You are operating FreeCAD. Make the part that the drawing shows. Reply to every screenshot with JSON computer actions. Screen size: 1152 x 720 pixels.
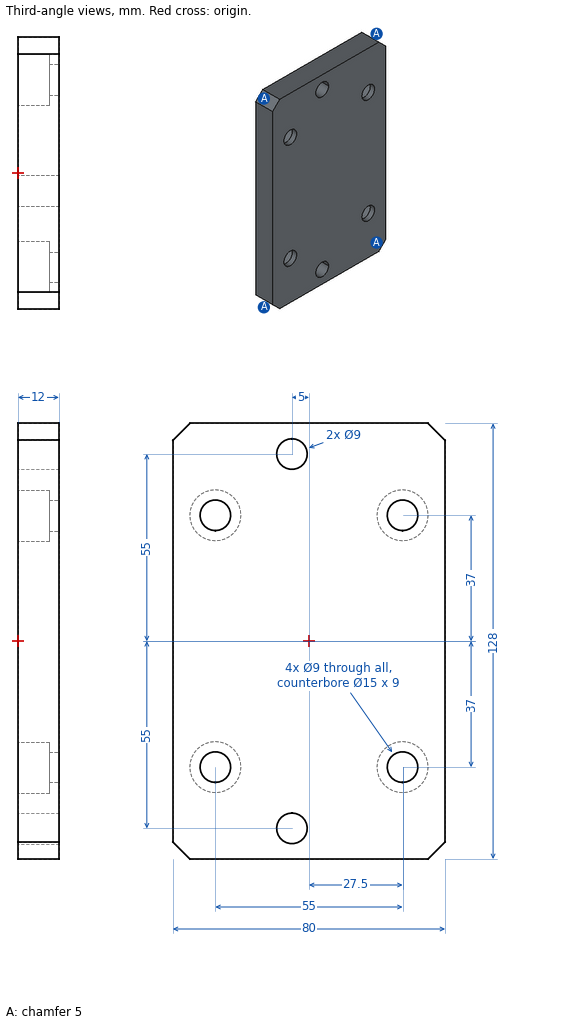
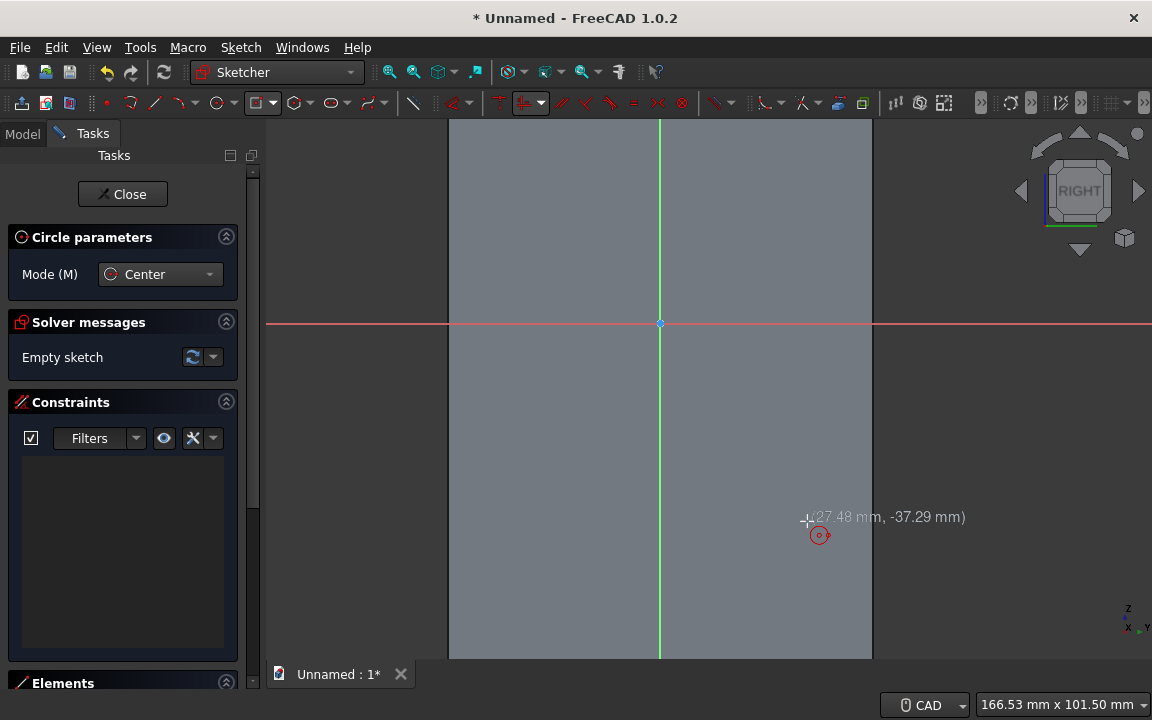
{"action": "left_click", "coordinate": [807, 521]}
{"action": "left_click", "coordinate": [824, 504]}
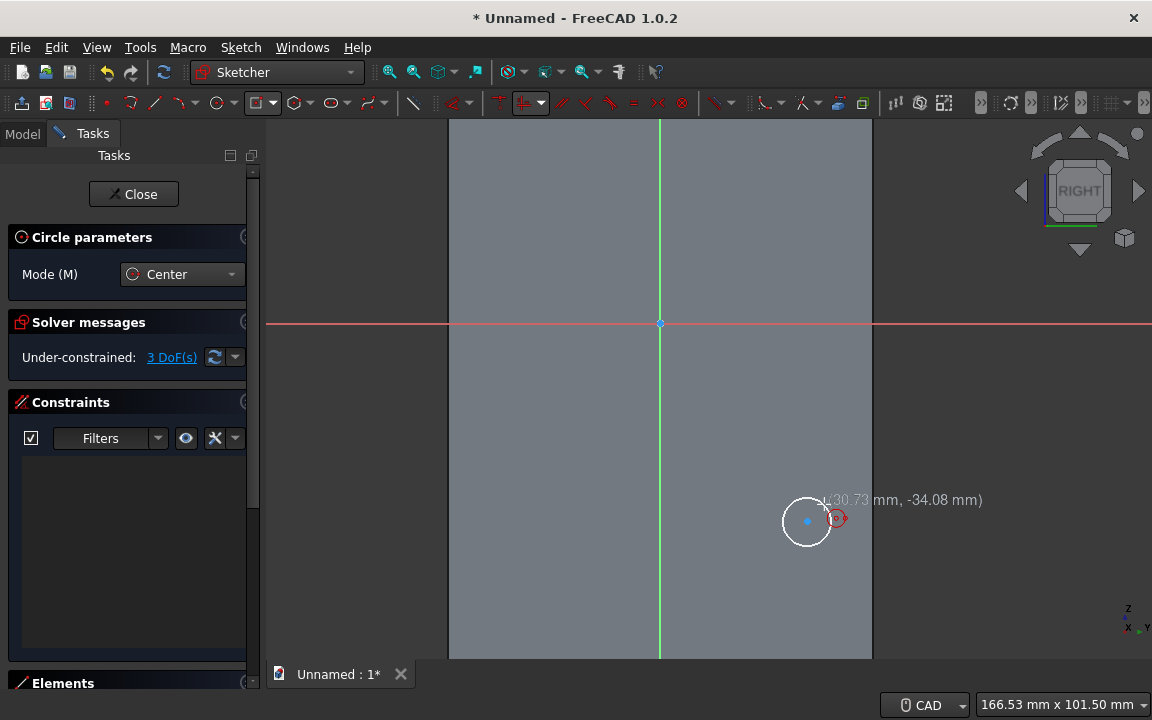
{"action": "left_click", "coordinate": [514, 521]}
{"action": "left_click", "coordinate": [531, 504]}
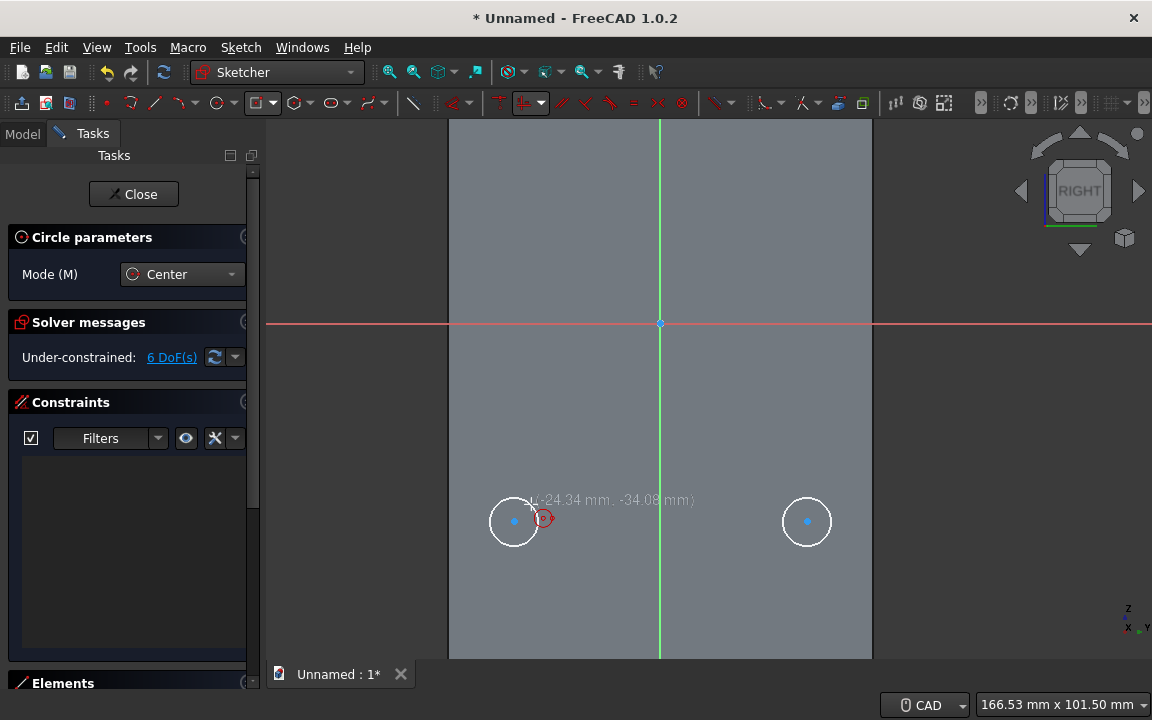
{"action": "scroll", "coordinate": [550, 631], "scroll_direction": "down", "scroll_amount": 1}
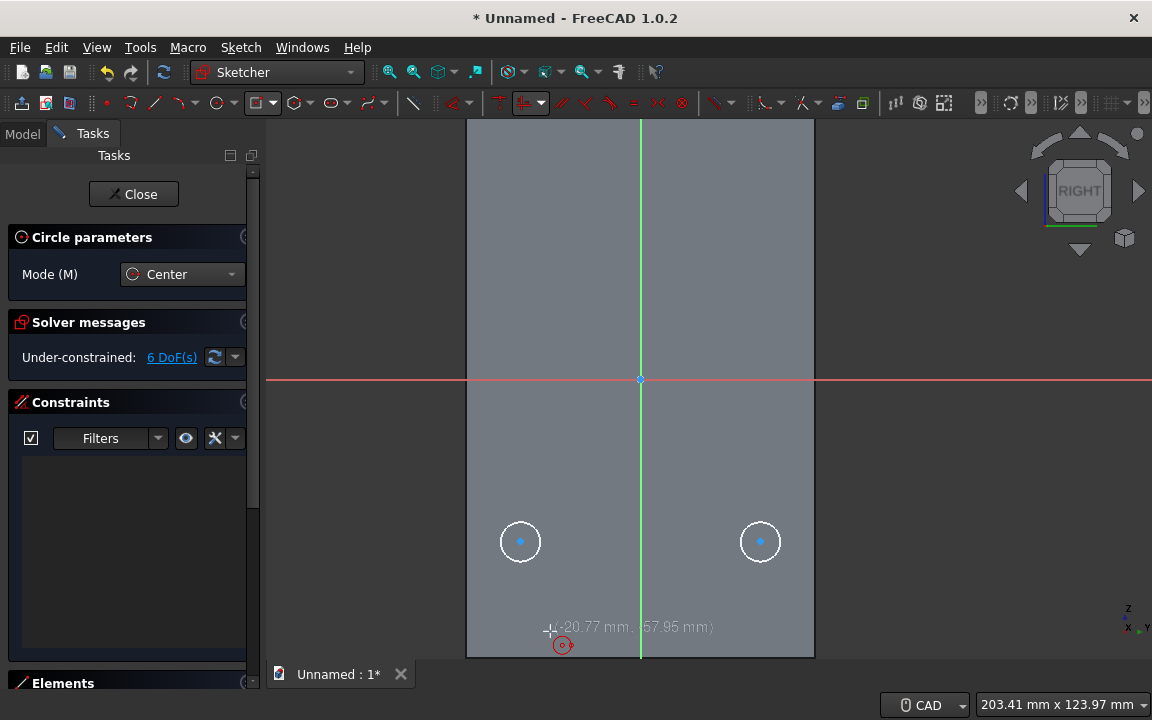
{"action": "left_click", "coordinate": [760, 218]}
{"action": "left_click", "coordinate": [774, 205]}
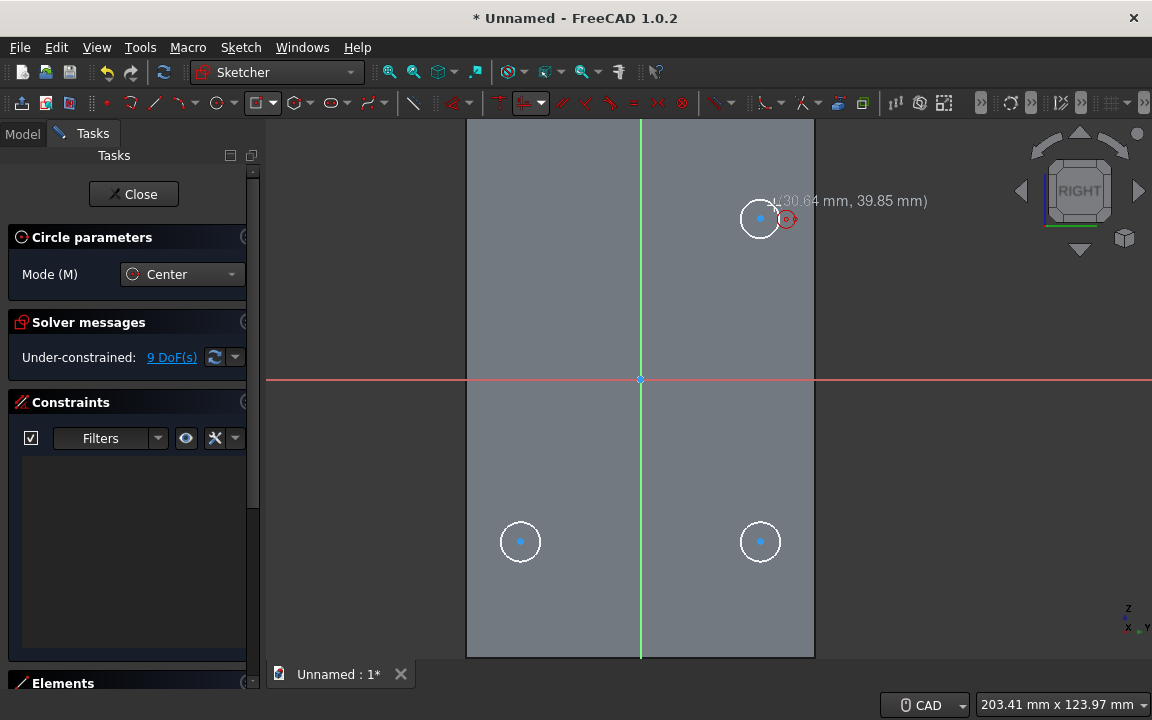
{"action": "left_click", "coordinate": [521, 218]}
{"action": "left_click", "coordinate": [535, 205]}
{"action": "key", "text": "Escape"}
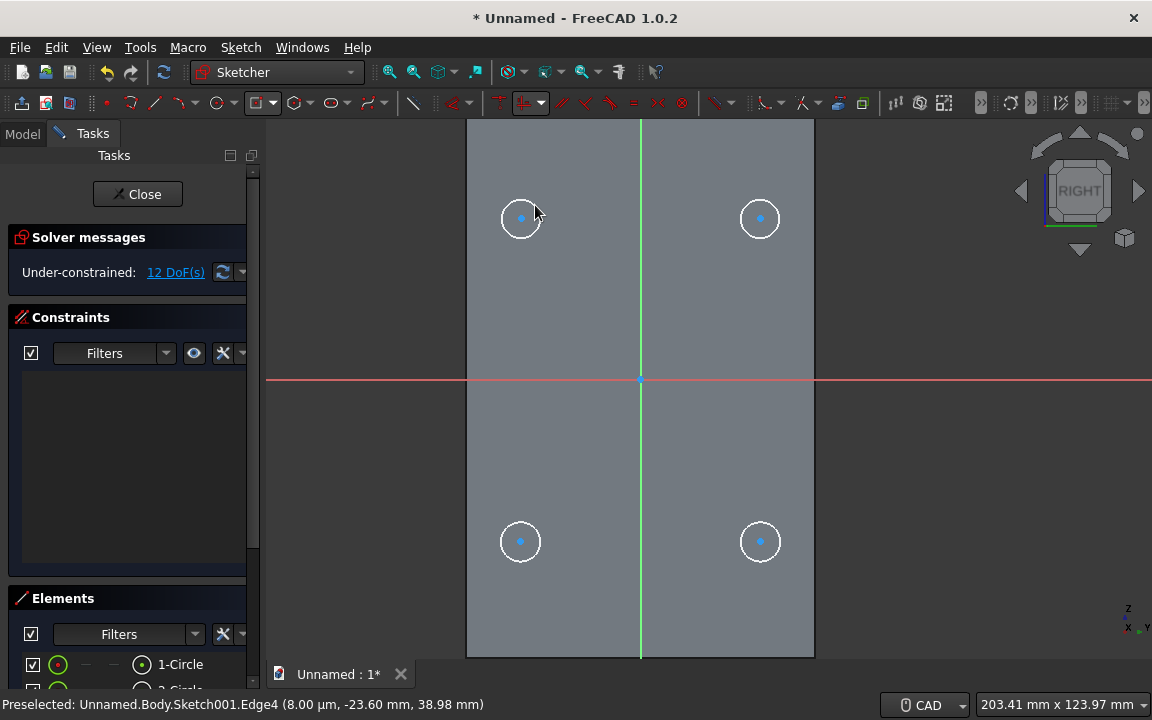
{"action": "left_click", "coordinate": [774, 528]}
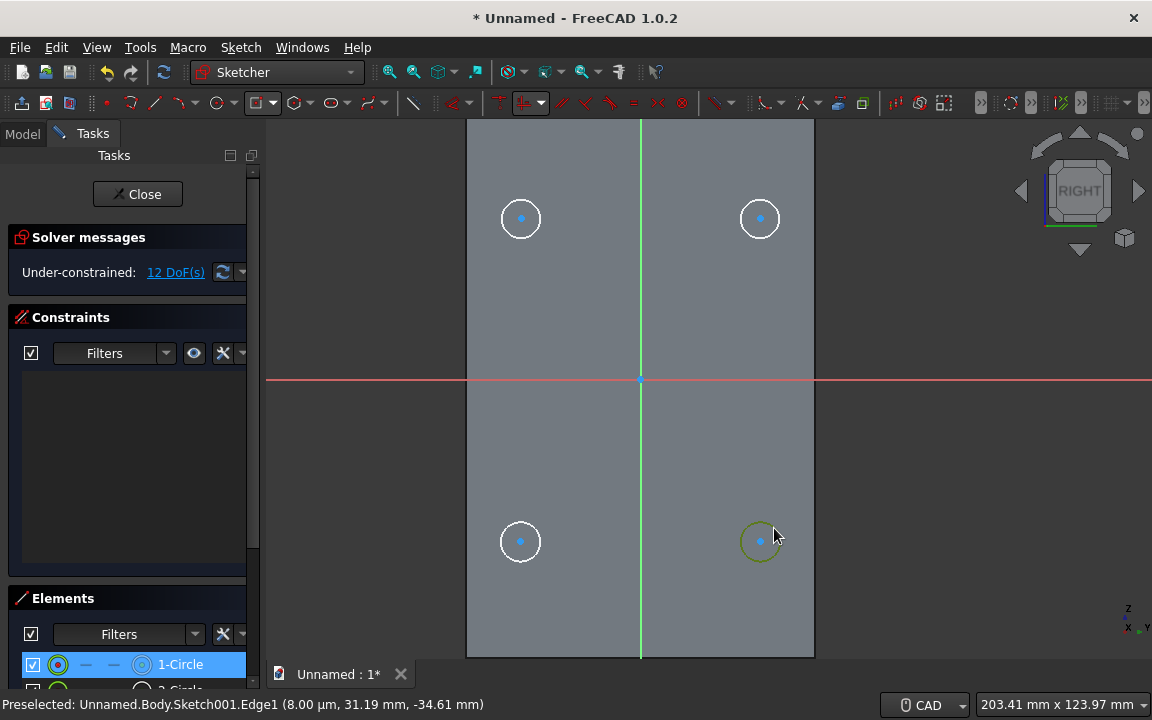
{"action": "left_click", "coordinate": [534, 528]}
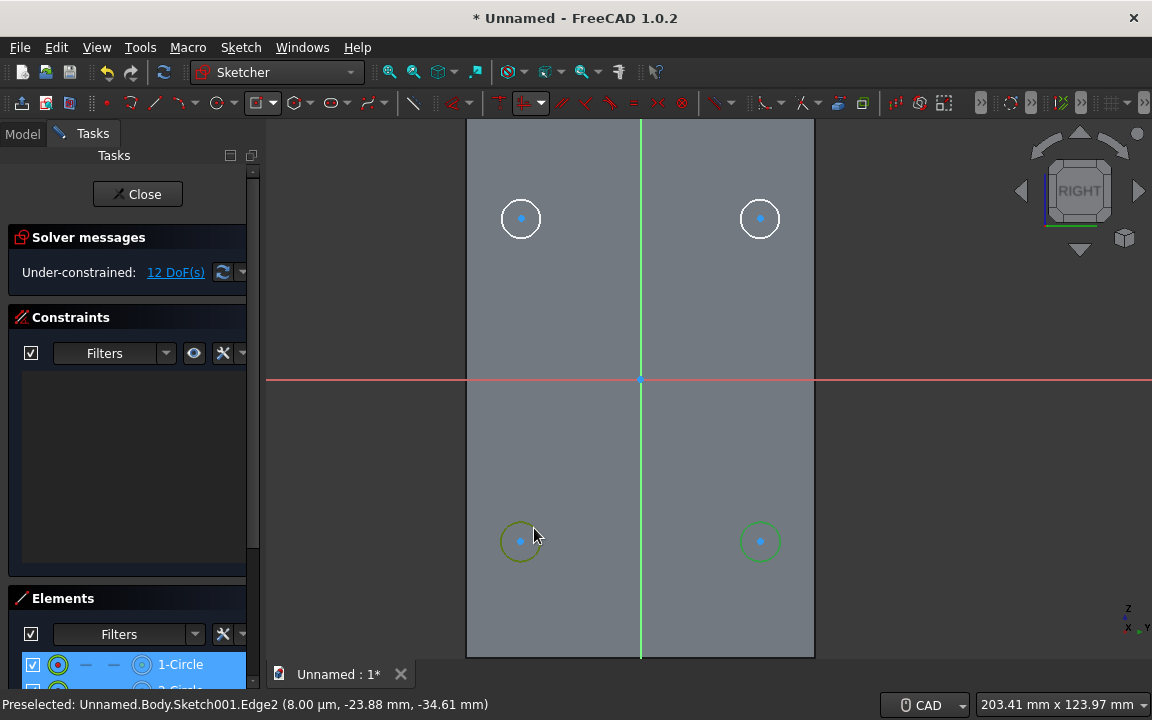
{"action": "left_click", "coordinate": [773, 205]}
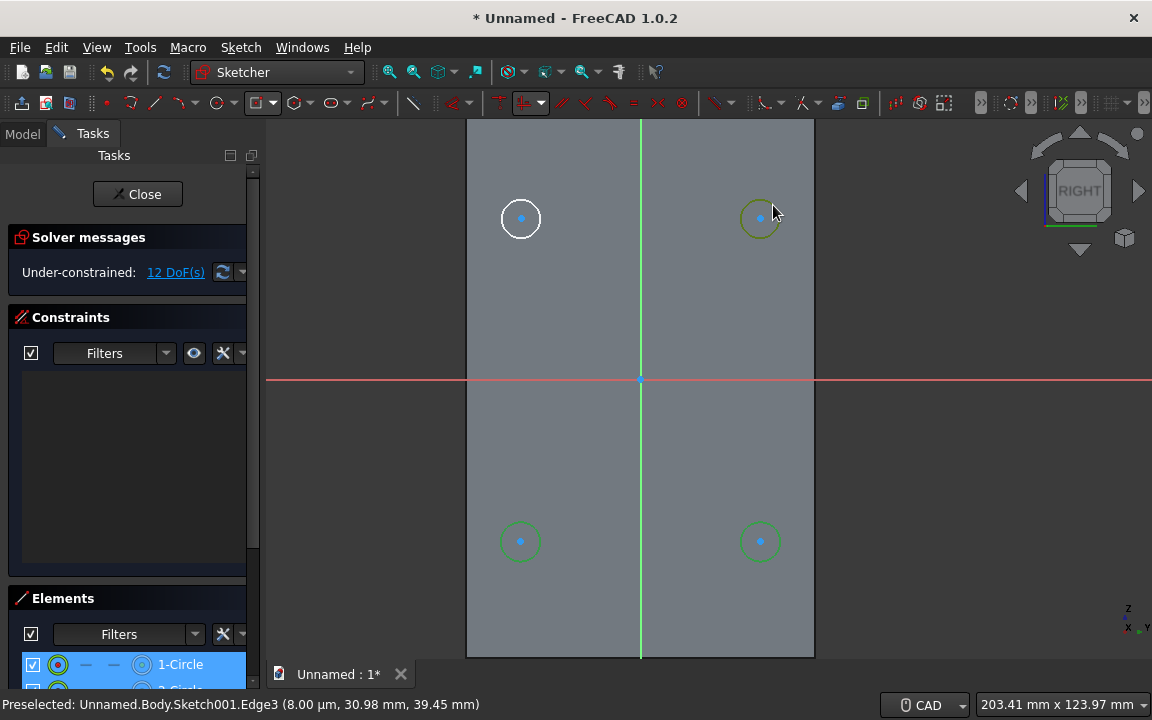
{"action": "left_click", "coordinate": [534, 205]}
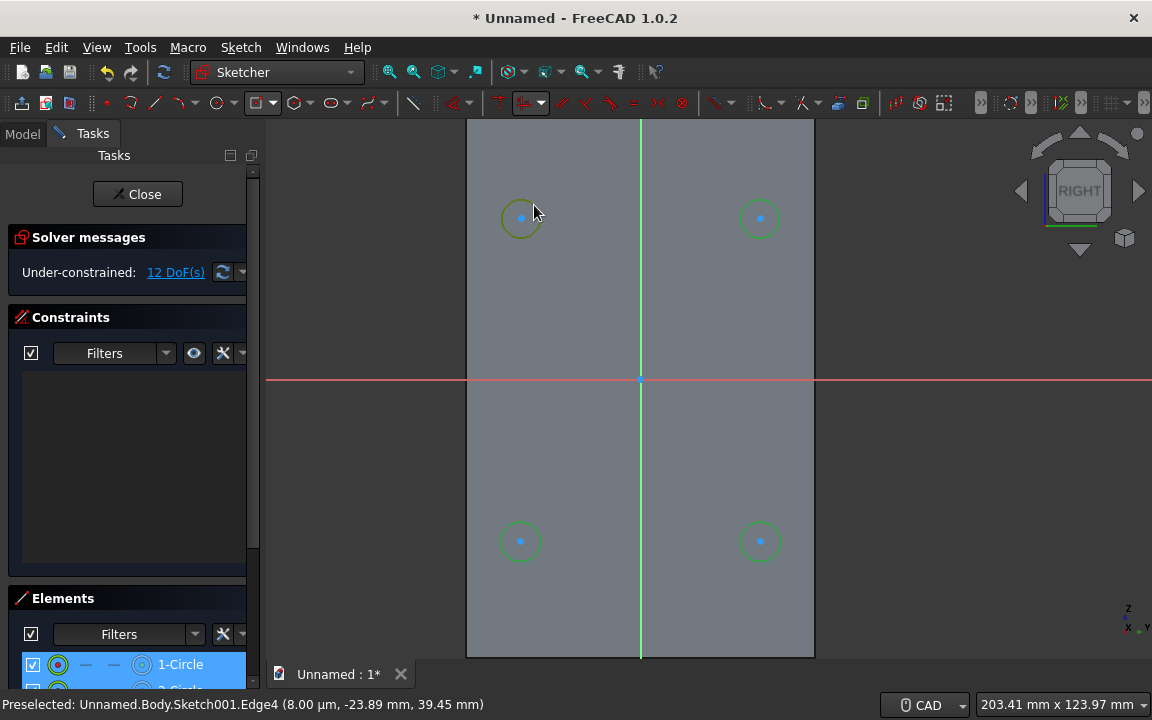
{"action": "left_click", "coordinate": [634, 104]}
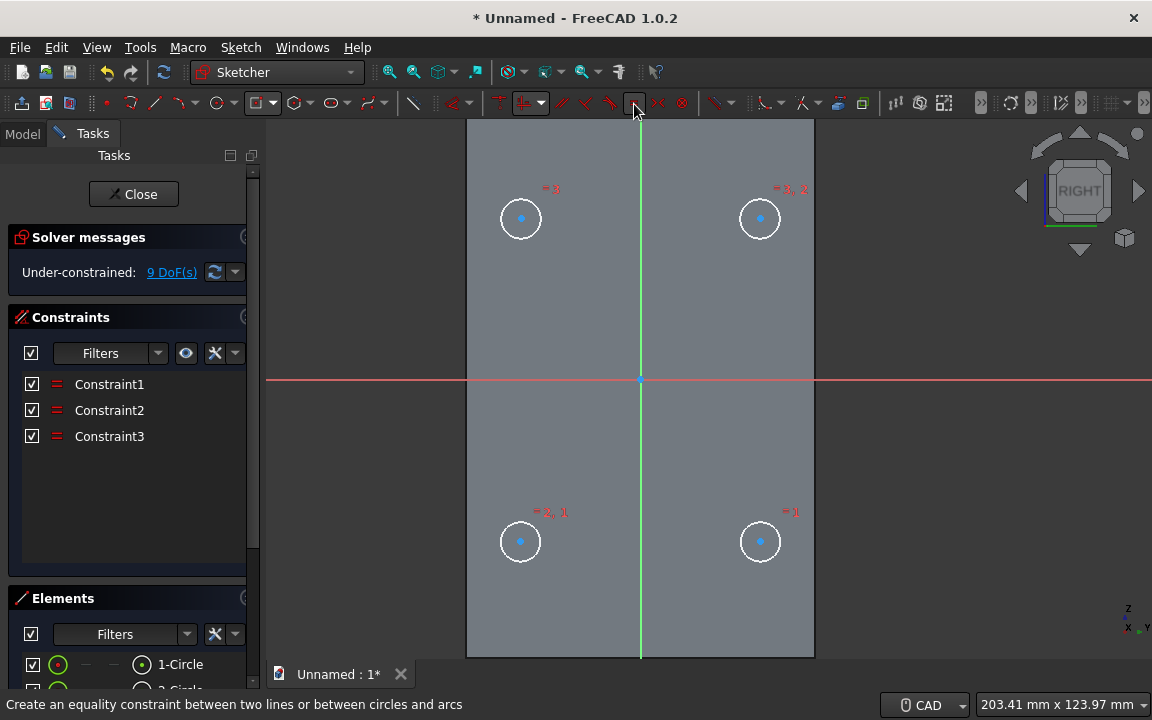
{"action": "left_click", "coordinate": [760, 542]}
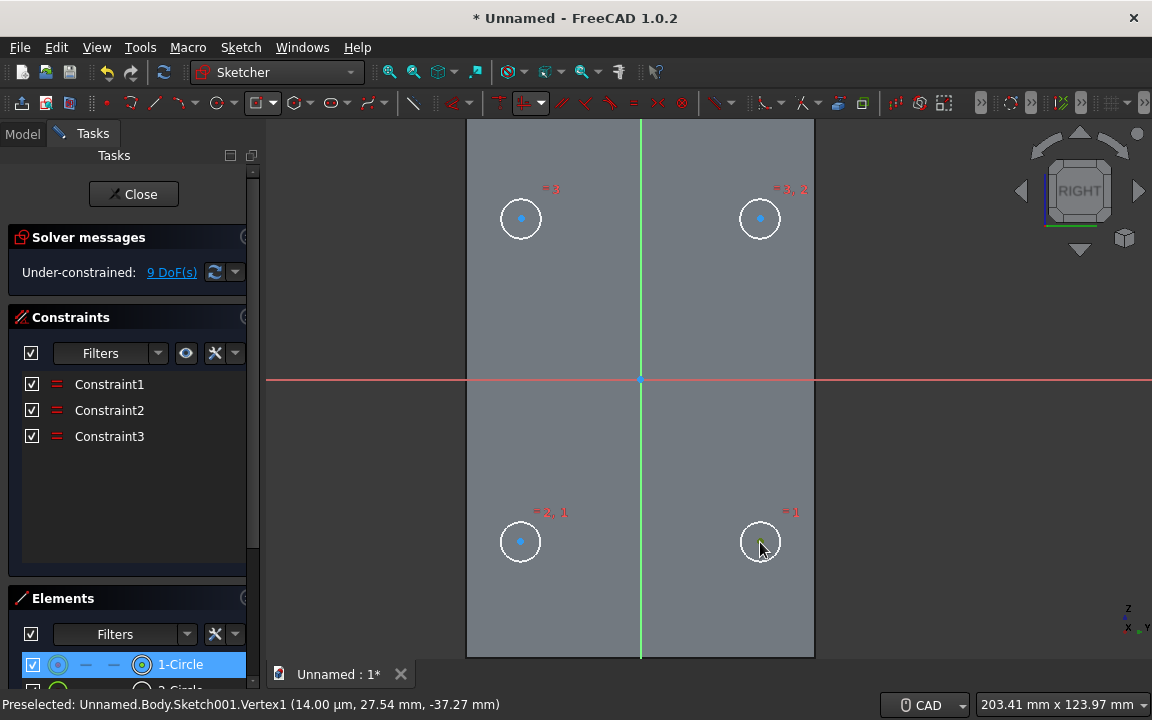
{"action": "left_click", "coordinate": [521, 542]}